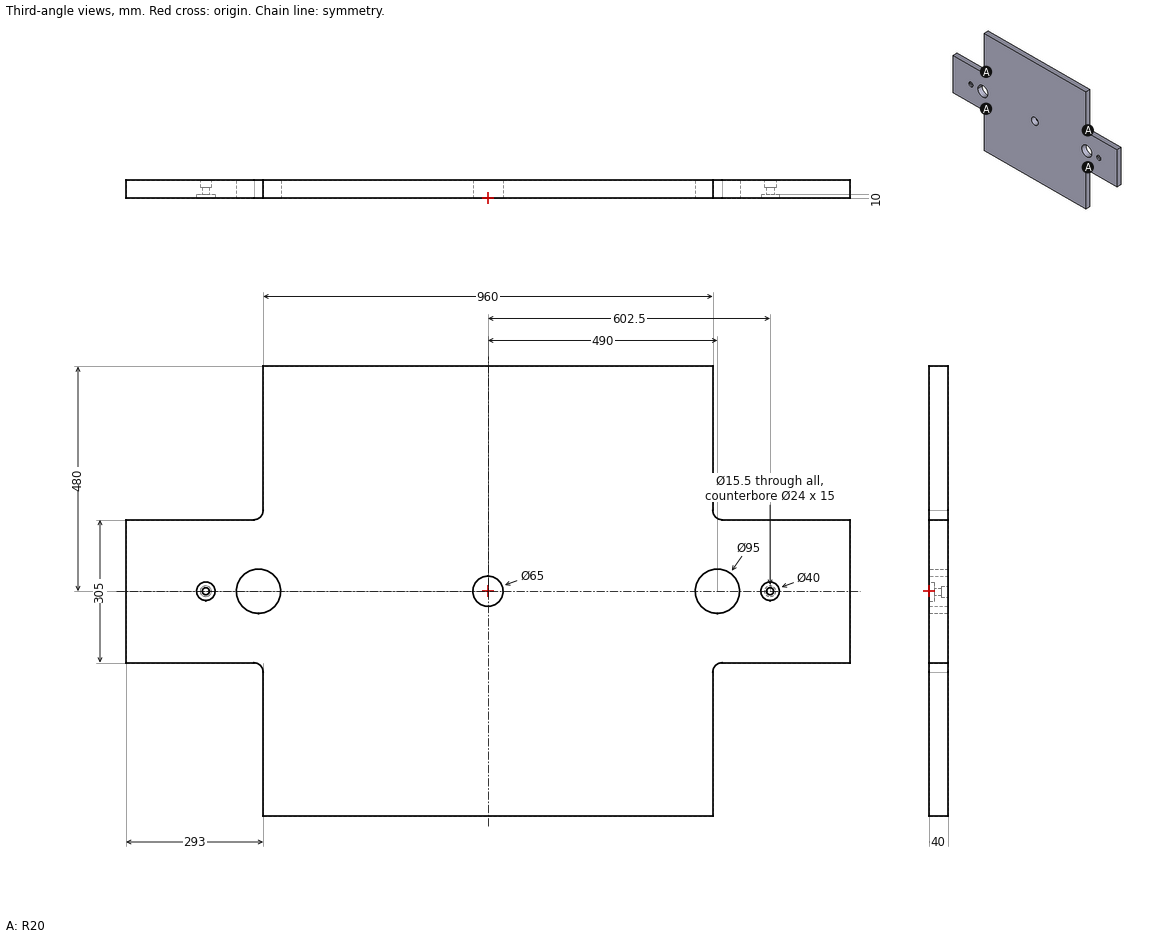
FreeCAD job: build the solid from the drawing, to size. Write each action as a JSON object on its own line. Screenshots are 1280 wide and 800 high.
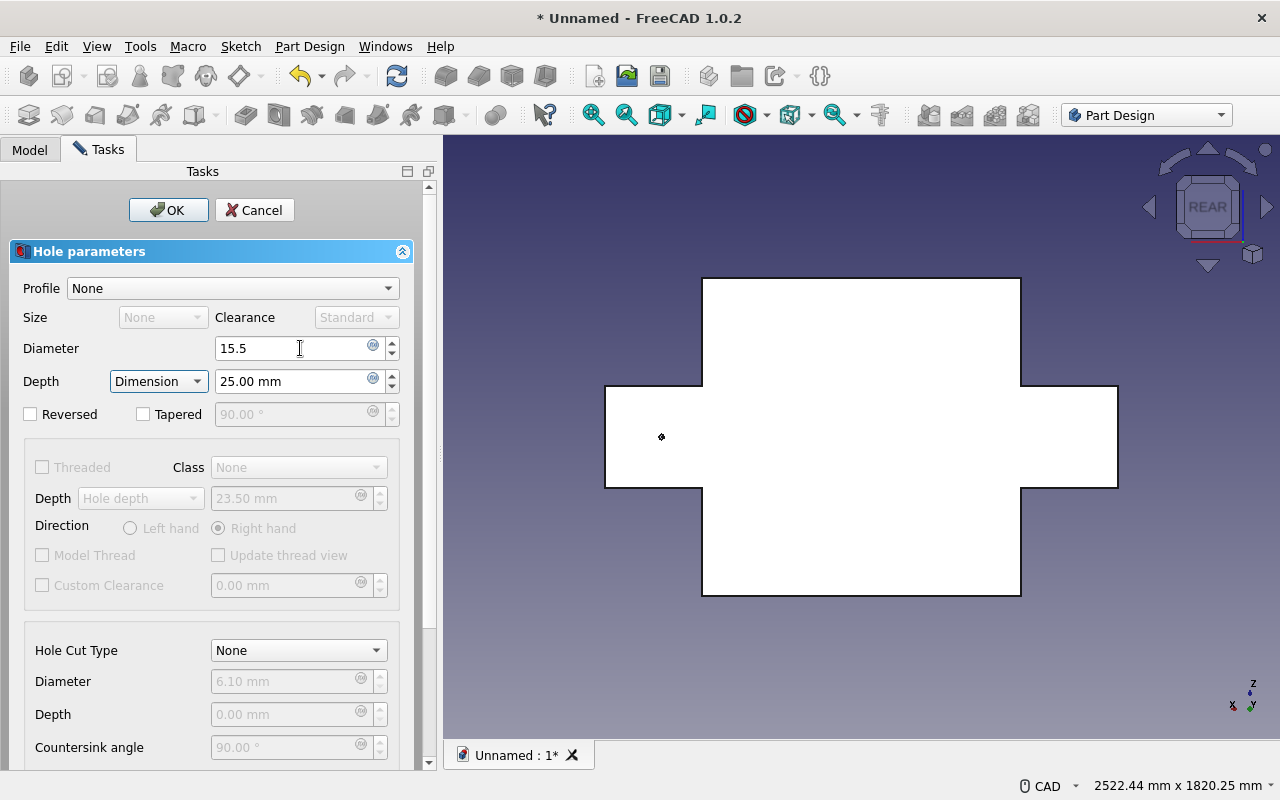
{"action": "left_click", "coordinate": [160, 382]}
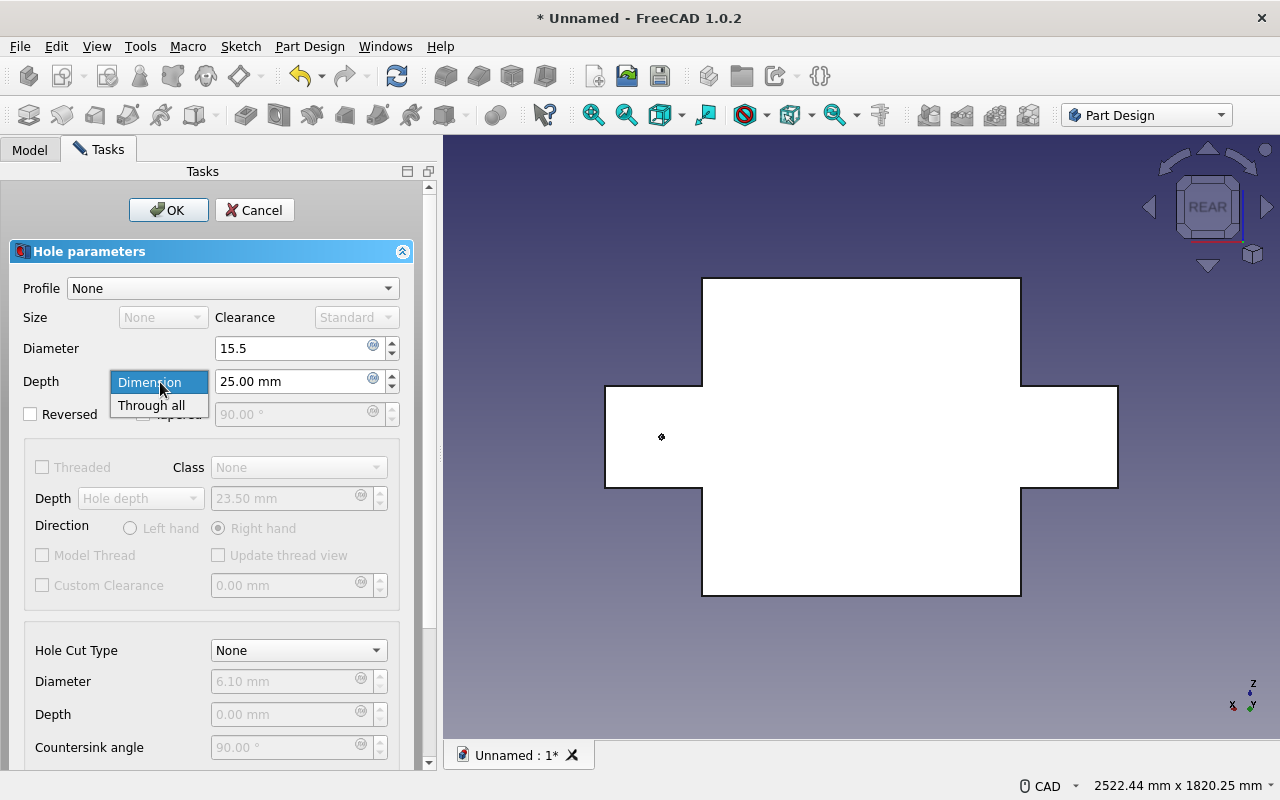
{"action": "left_click", "coordinate": [158, 406]}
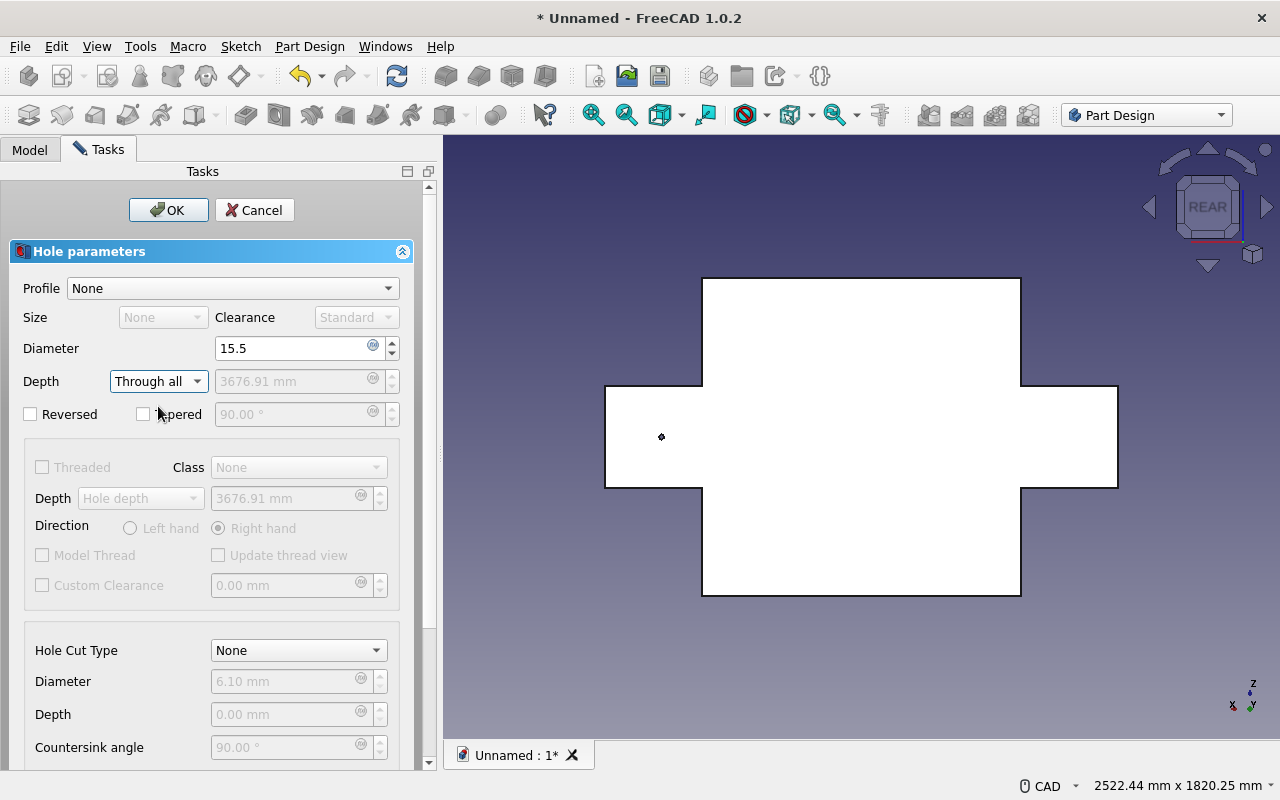
{"action": "left_click", "coordinate": [300, 650]}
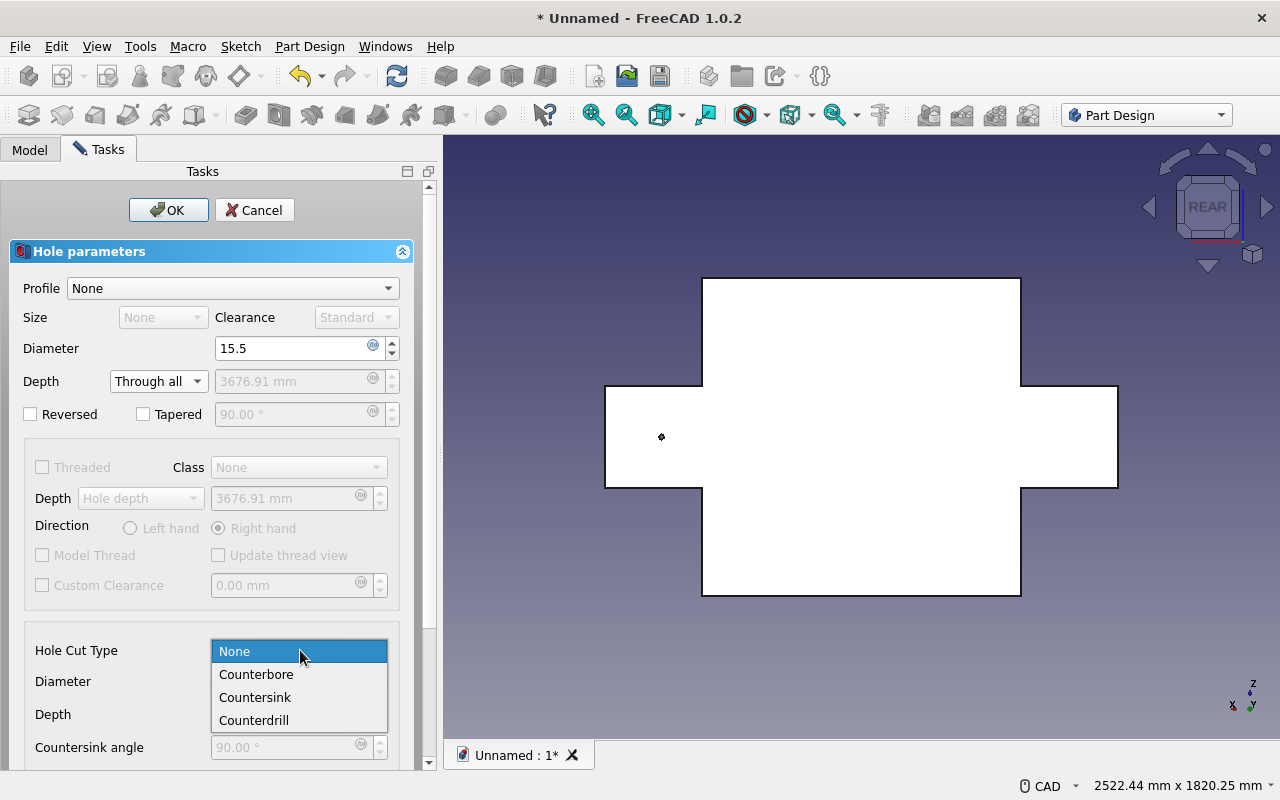
{"action": "left_click", "coordinate": [298, 674]}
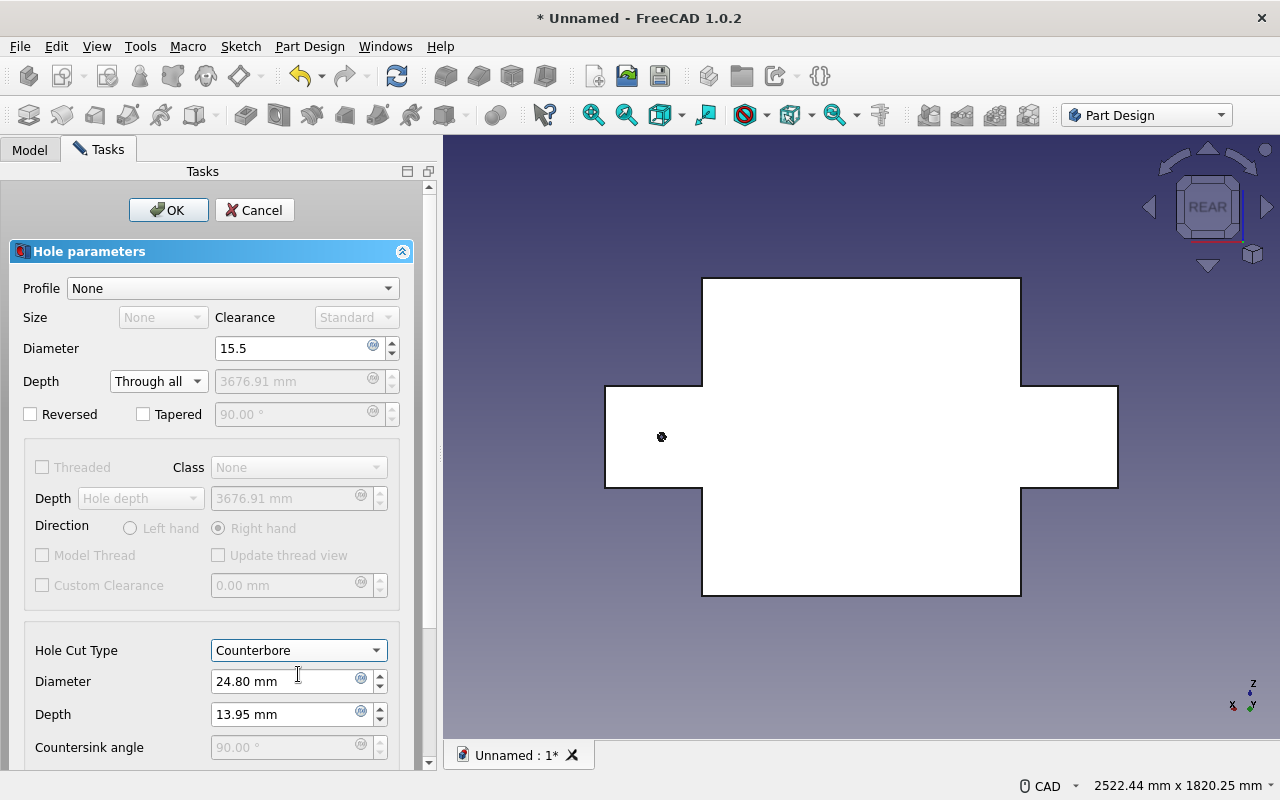
{"action": "triple_click", "coordinate": [292, 682]}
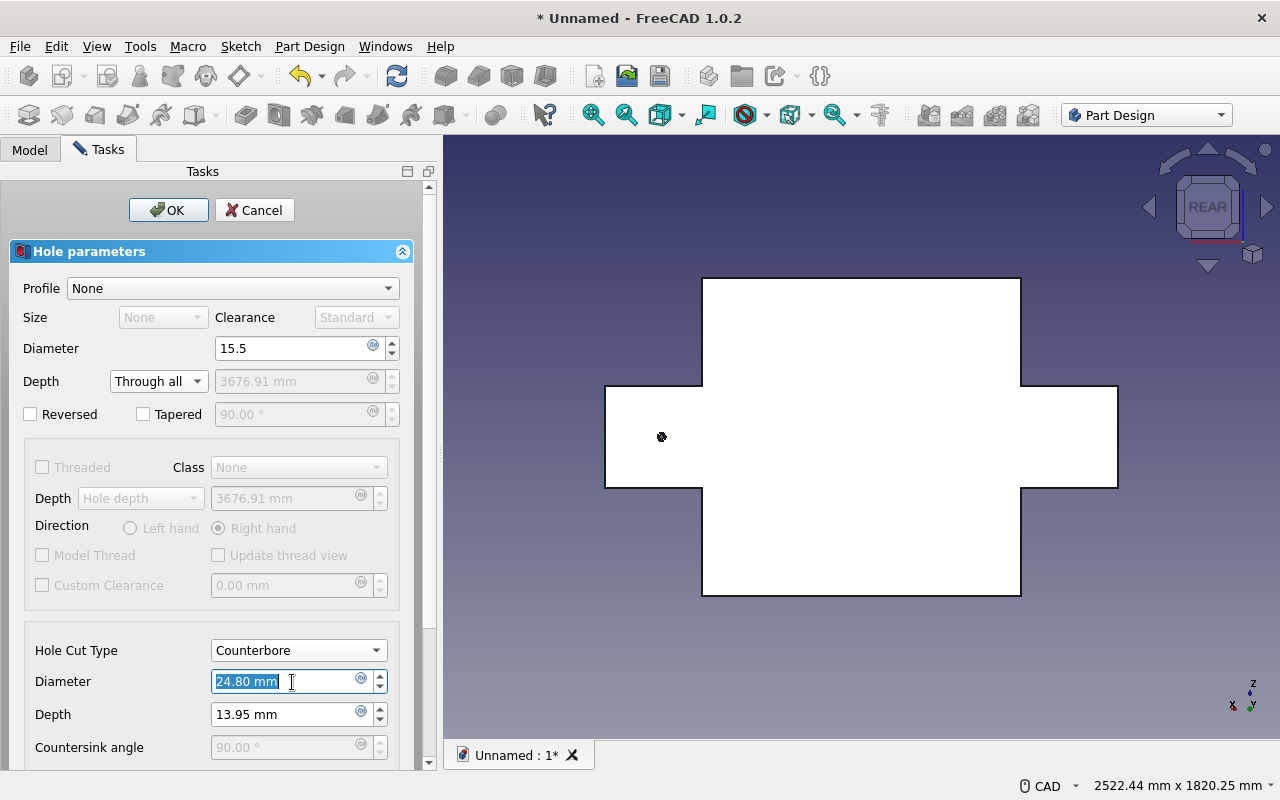
{"action": "type", "text": "24"}
{"action": "key", "text": "Tab"}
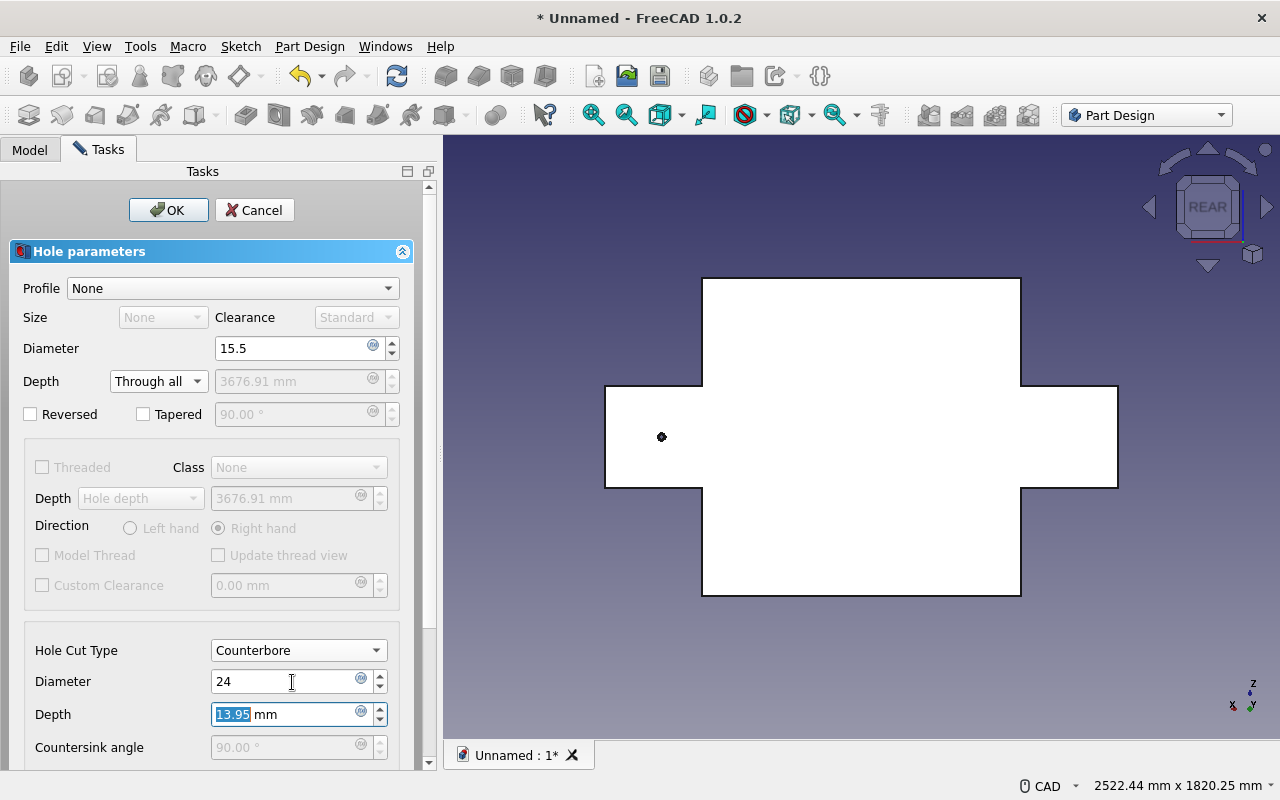
{"action": "type", "text": "15"}
{"action": "key", "text": "Tab"}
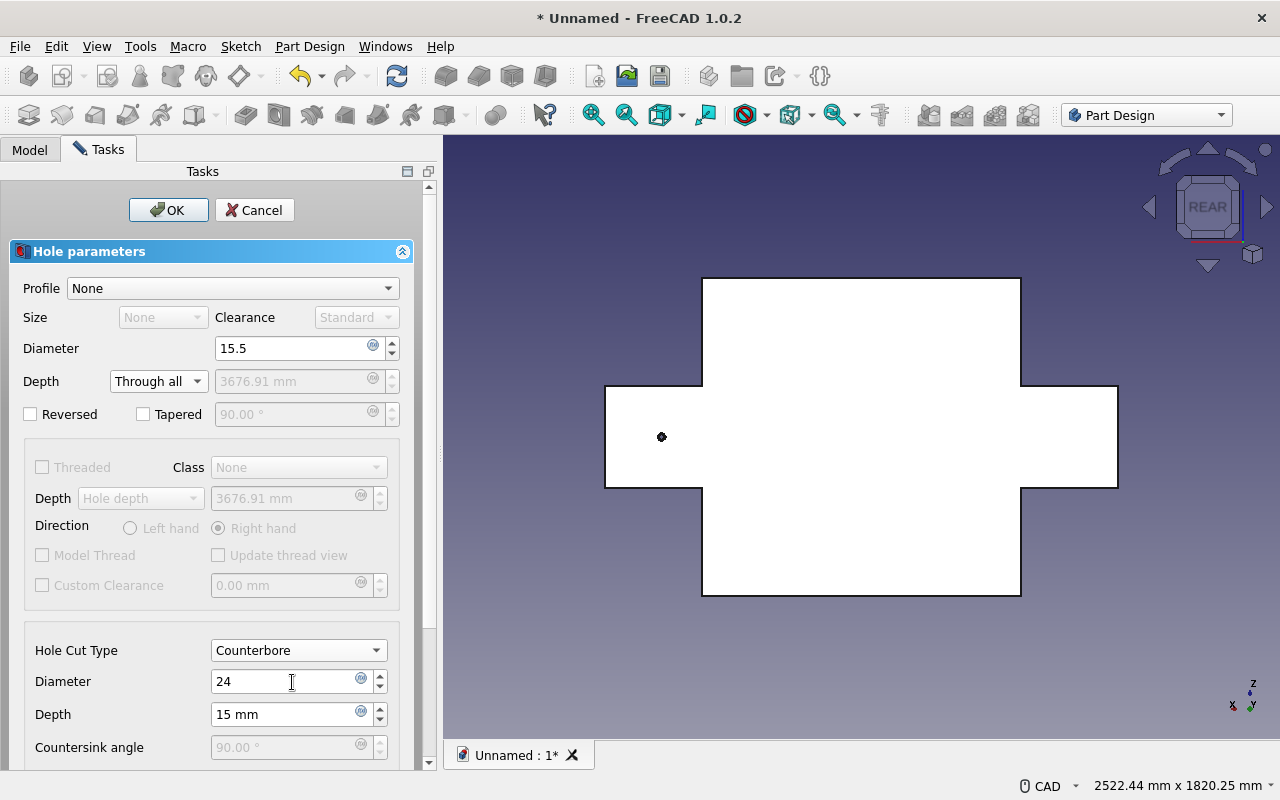
{"action": "left_click", "coordinate": [169, 210]}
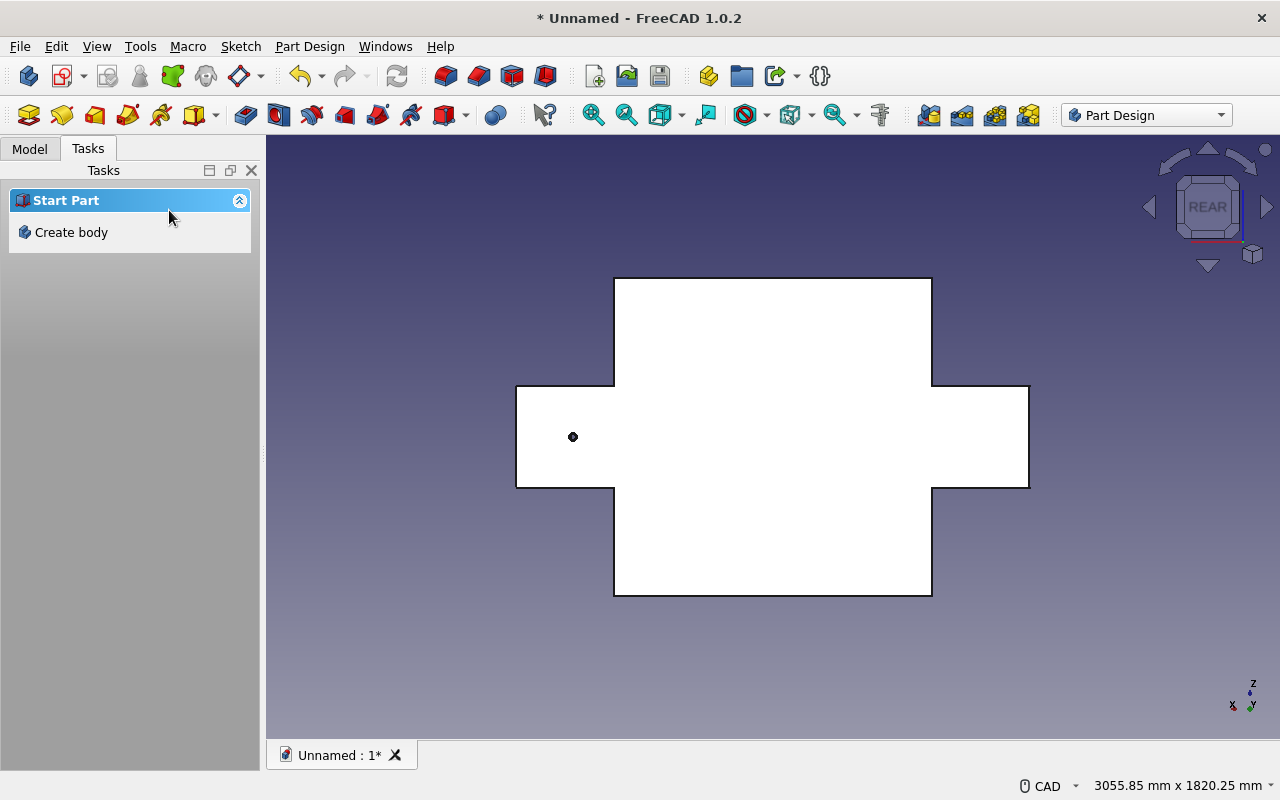
{"action": "left_click", "coordinate": [30, 148]}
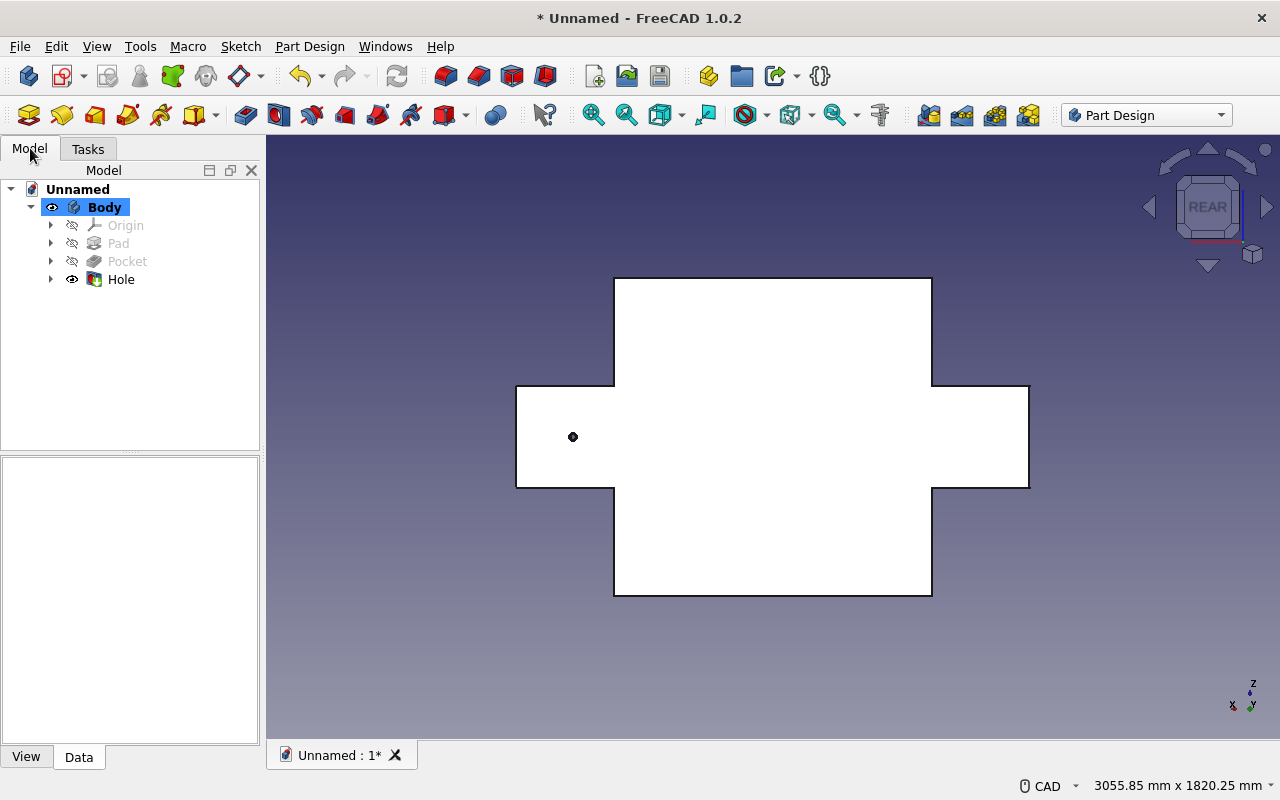
{"action": "left_click", "coordinate": [117, 261]}